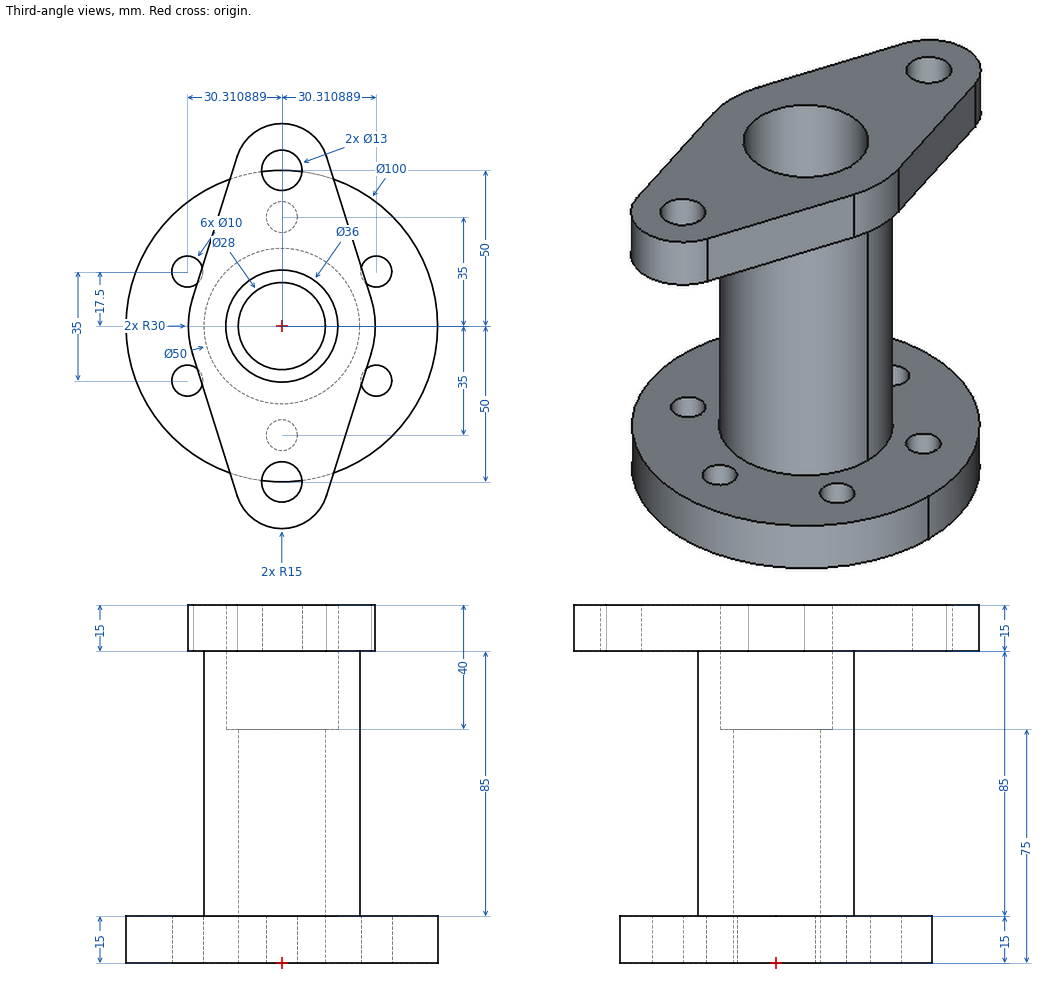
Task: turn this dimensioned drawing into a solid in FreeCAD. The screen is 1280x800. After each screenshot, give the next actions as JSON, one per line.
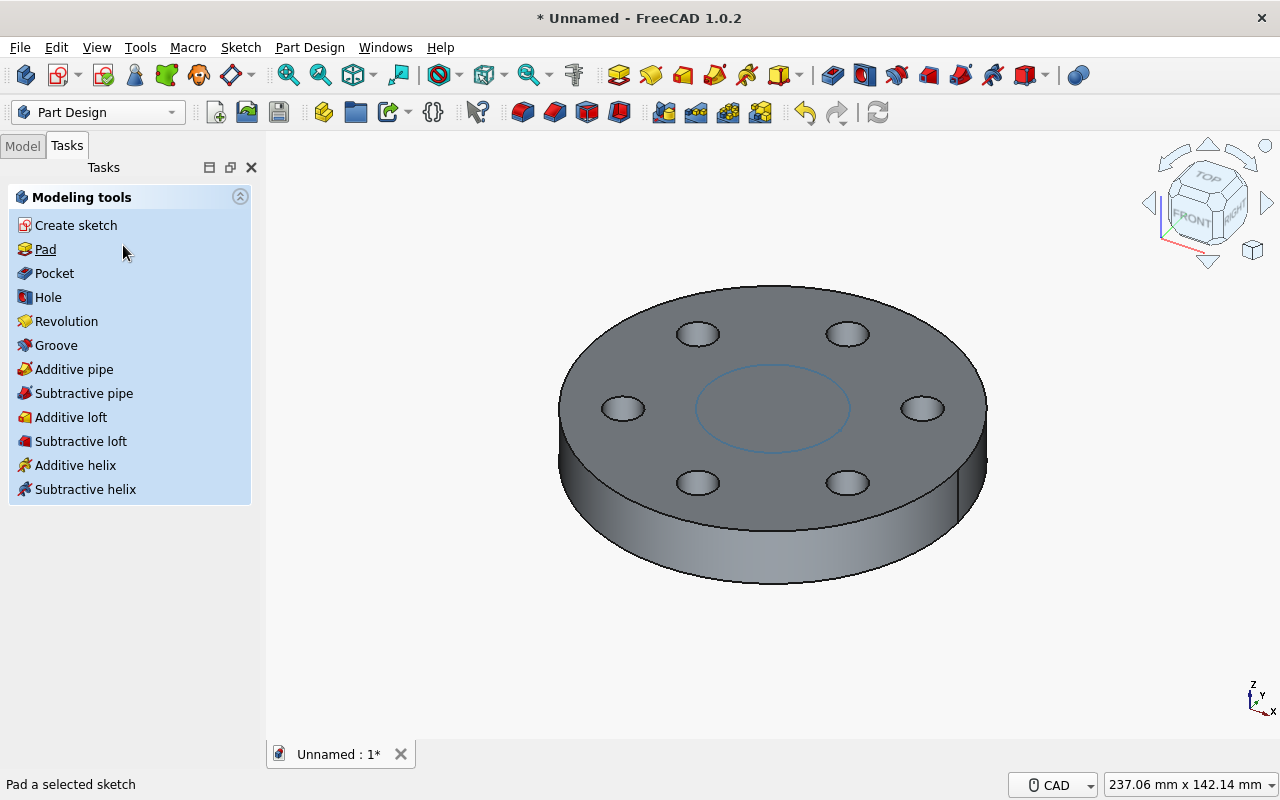
{"action": "left_click", "coordinate": [620, 76]}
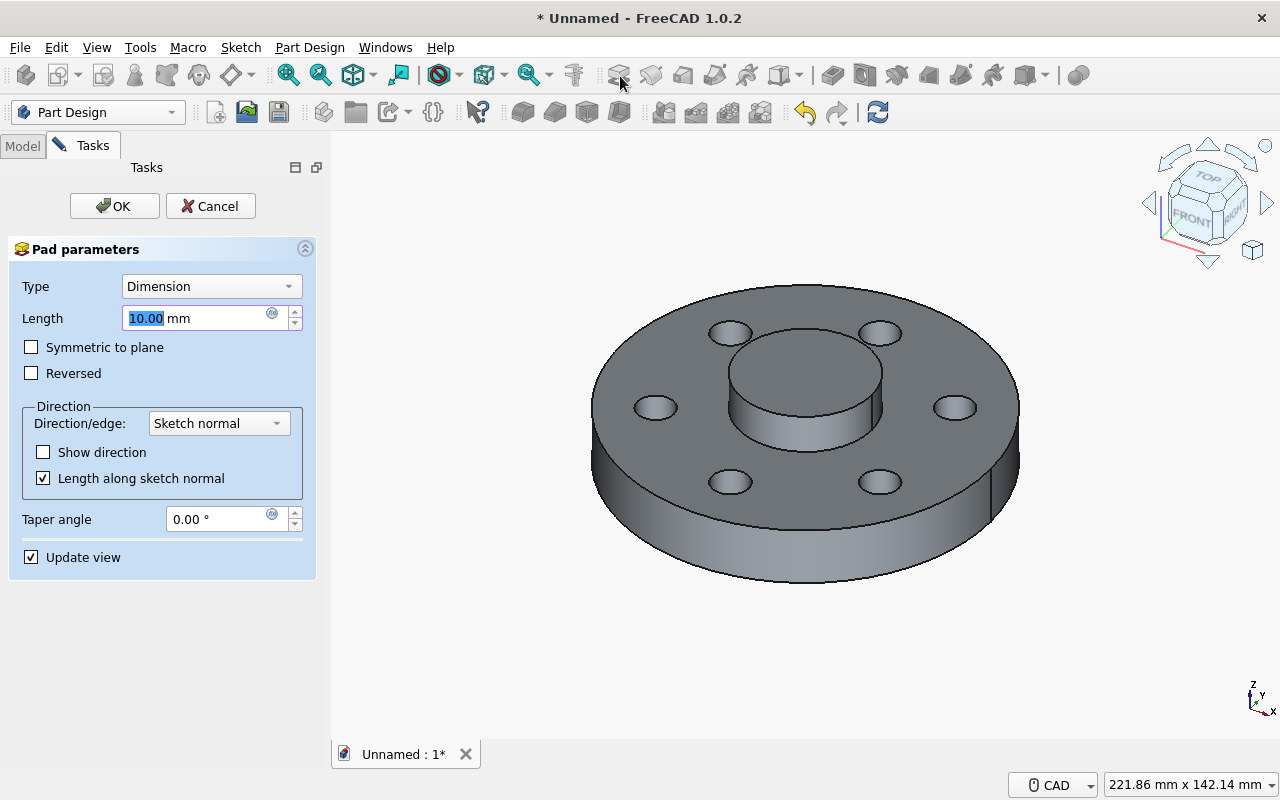
{"action": "type", "text": "85"}
{"action": "key", "text": "Tab"}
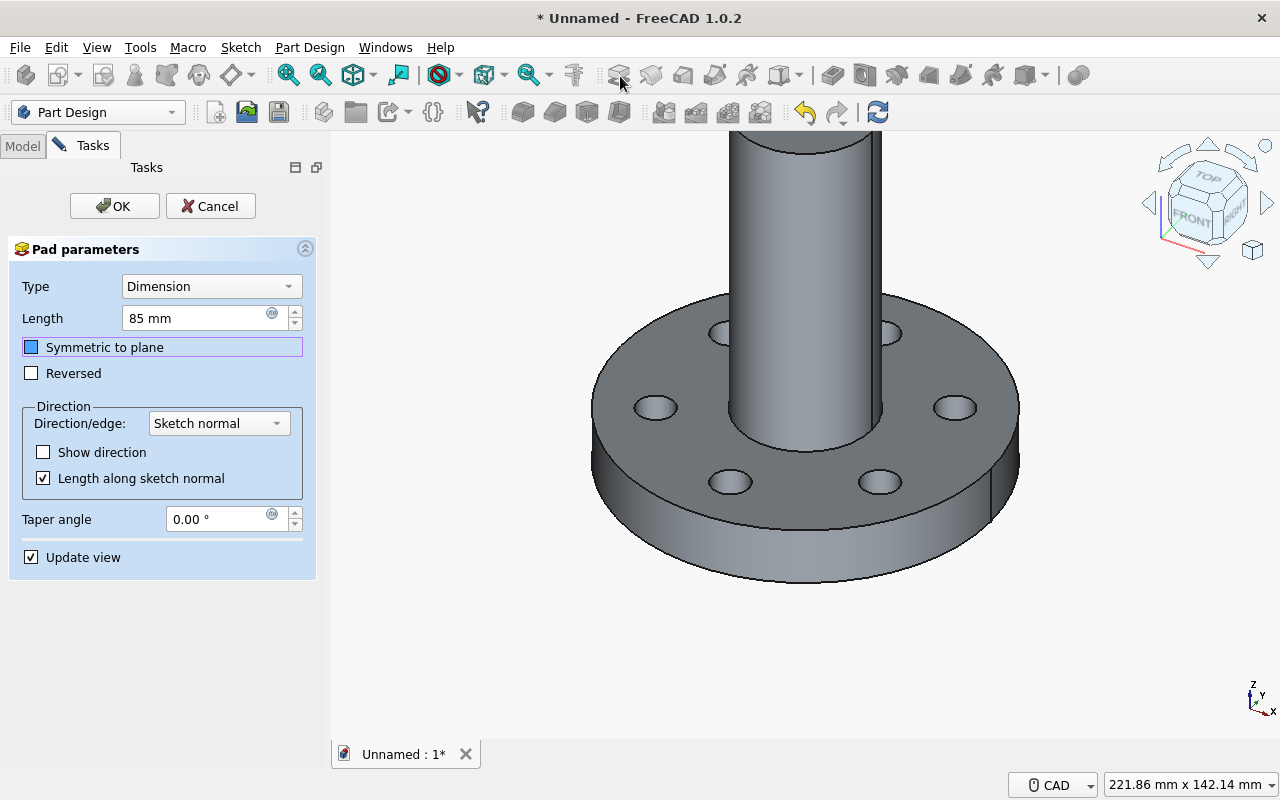
{"action": "left_click", "coordinate": [115, 206]}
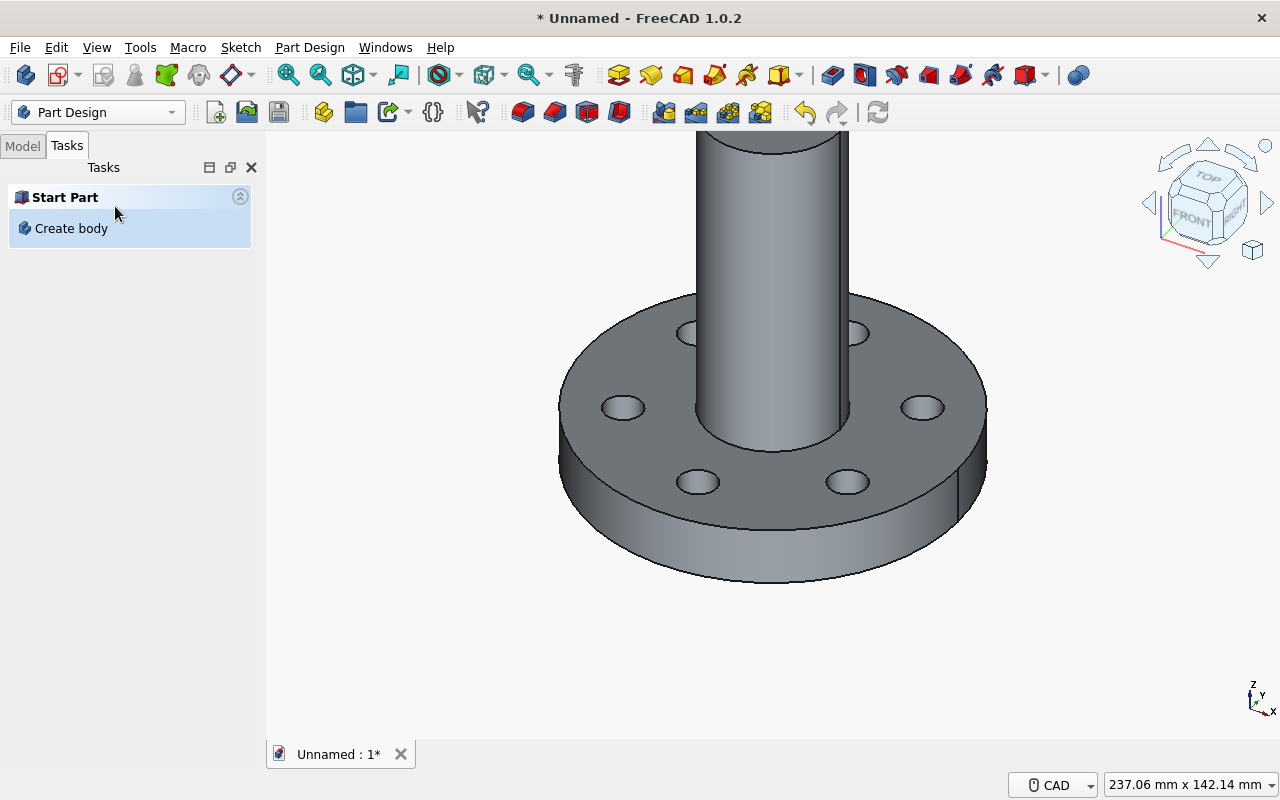
{"action": "key", "text": "v f"}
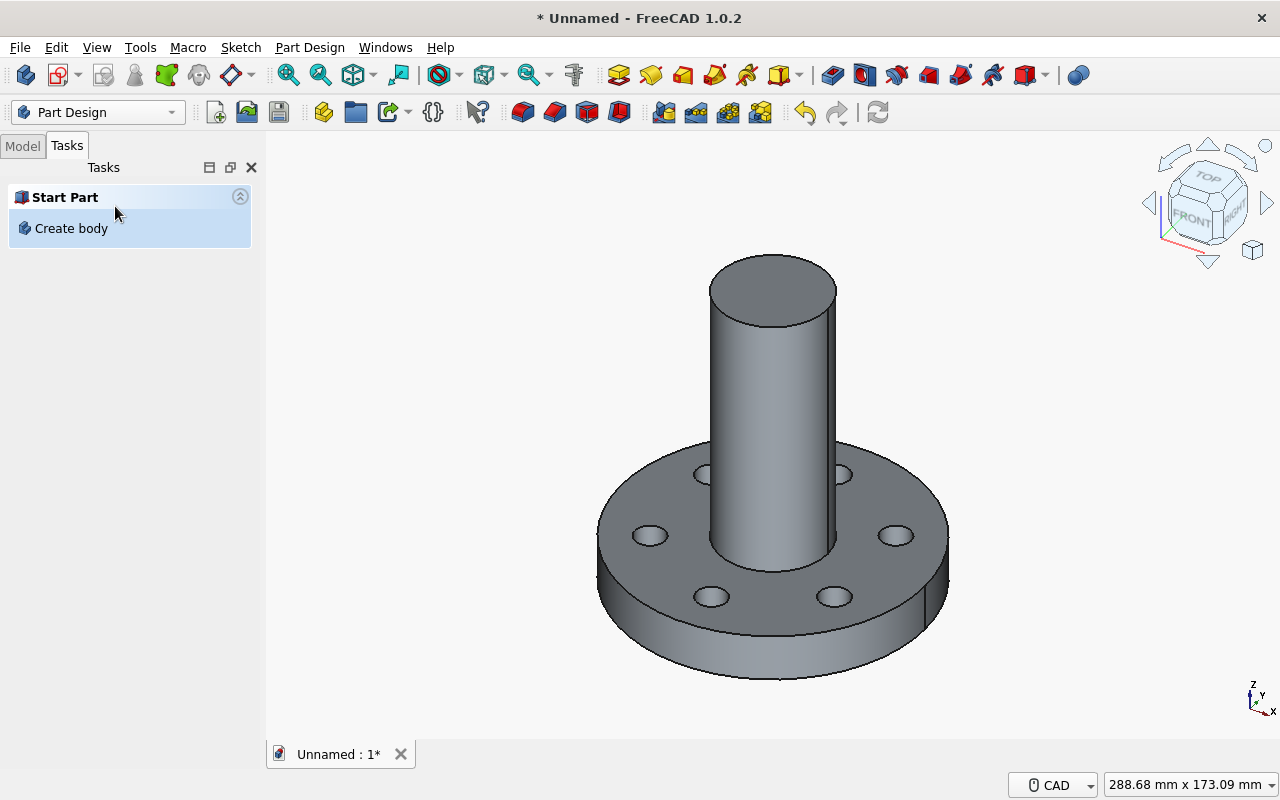
{"action": "left_click", "coordinate": [867, 499]}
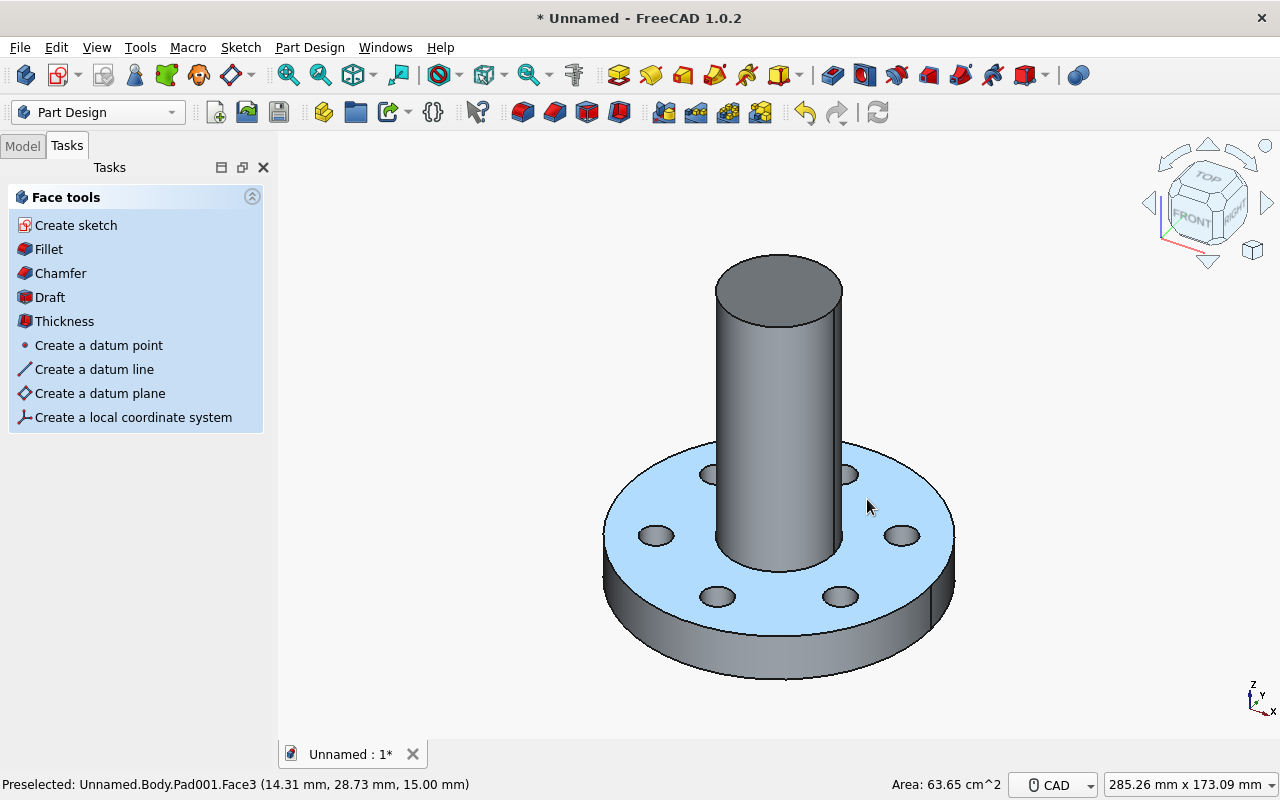
{"action": "left_click", "coordinate": [58, 76]}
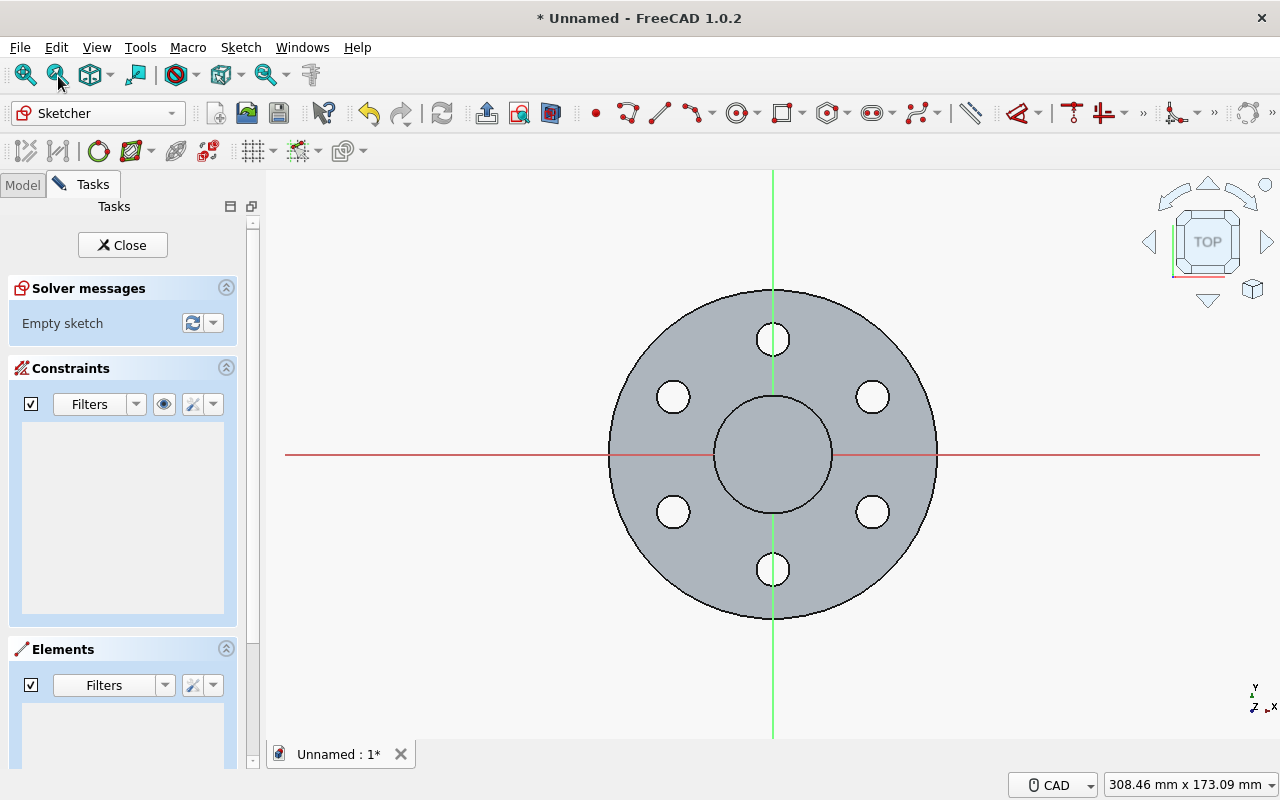
{"action": "key", "text": "q s"}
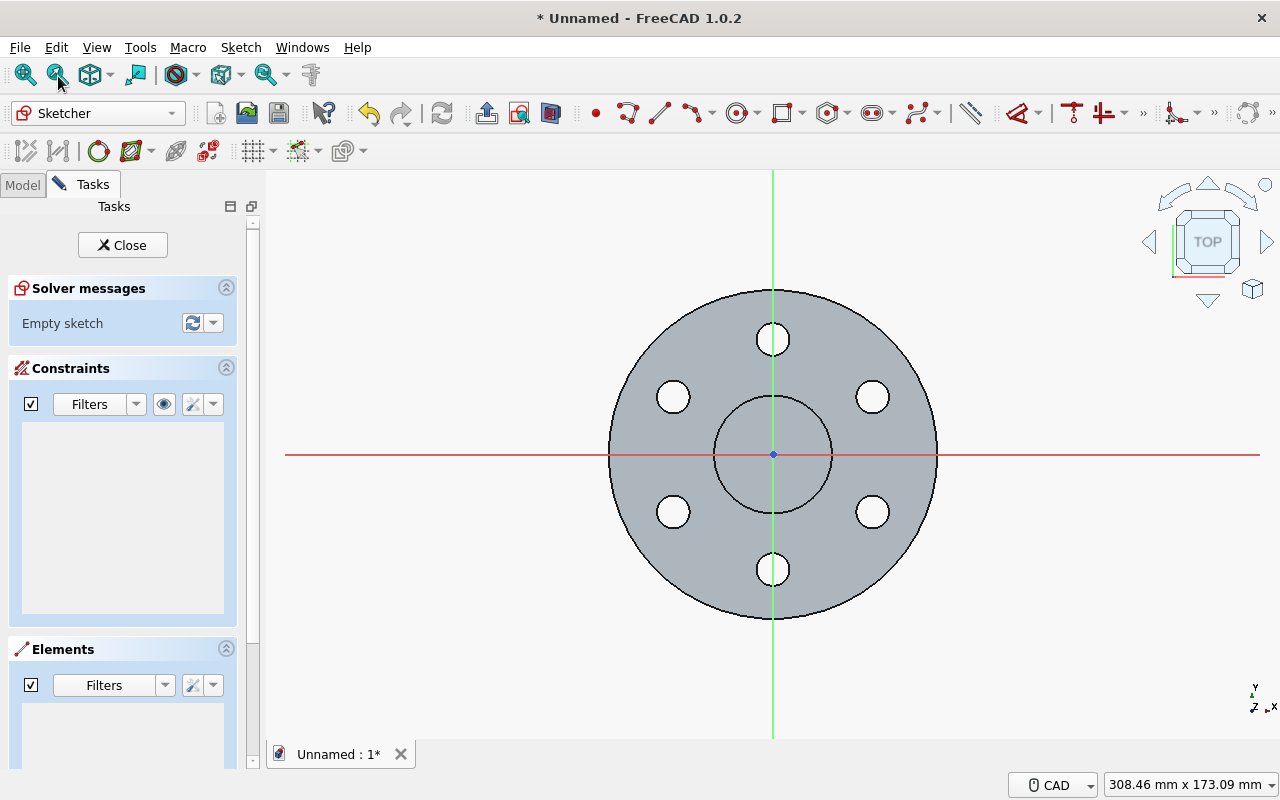
{"action": "scroll", "coordinate": [803, 455], "scroll_direction": "up", "scroll_amount": 6}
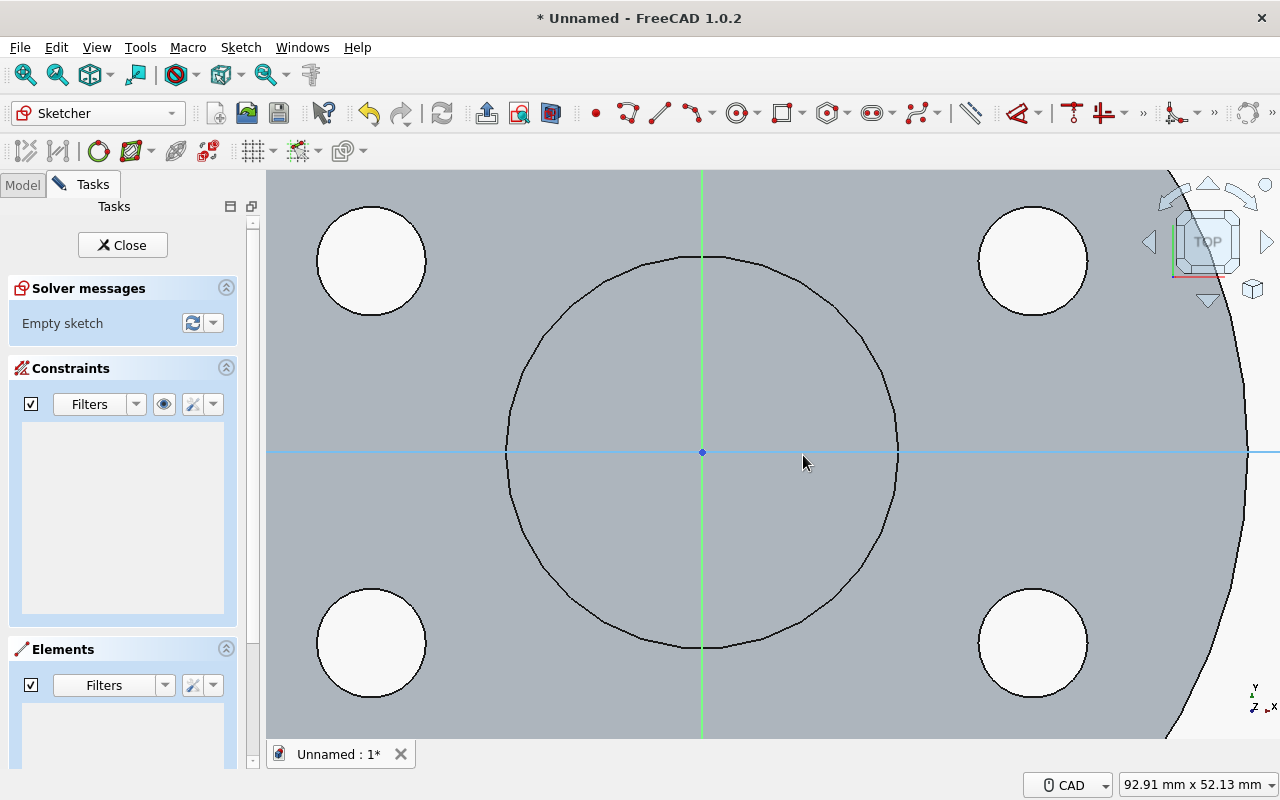
{"action": "key", "text": "g c"}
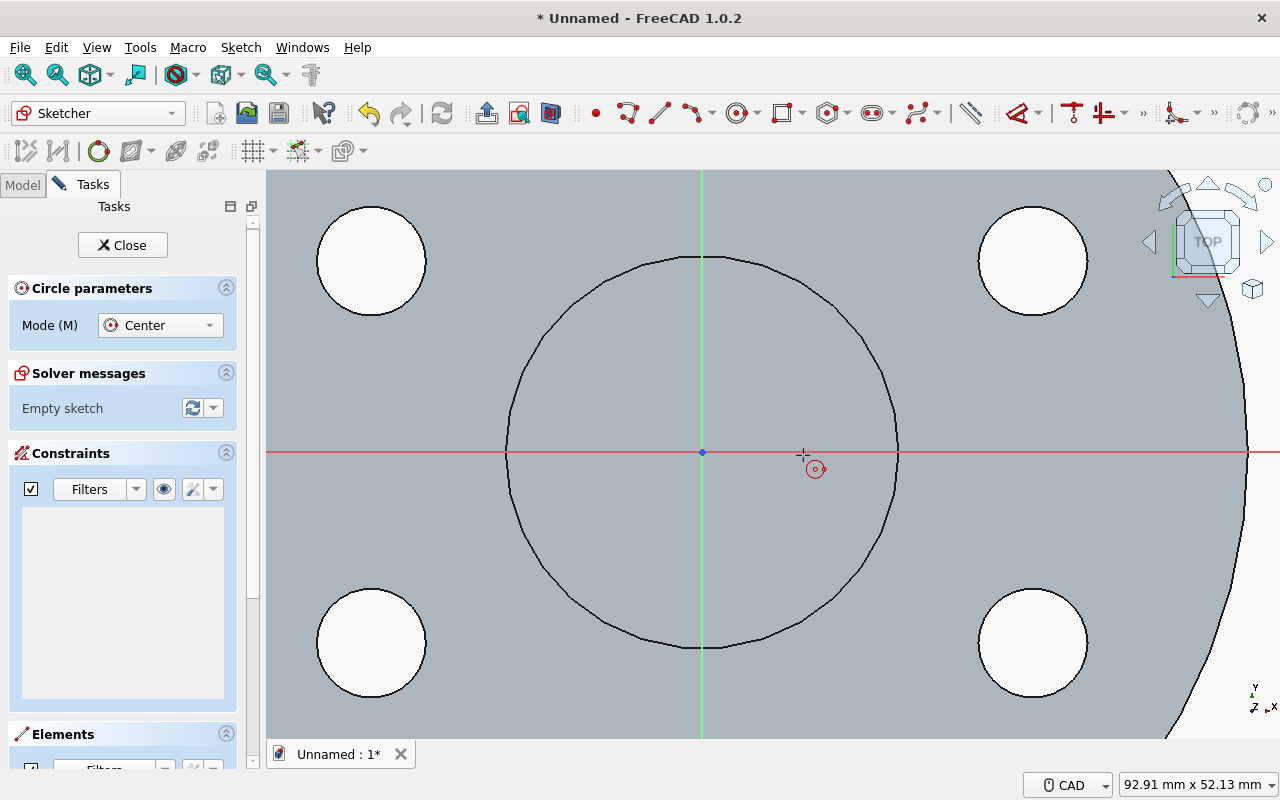
{"action": "left_click", "coordinate": [702, 452]}
{"action": "mouse_move", "coordinate": [841, 313]}